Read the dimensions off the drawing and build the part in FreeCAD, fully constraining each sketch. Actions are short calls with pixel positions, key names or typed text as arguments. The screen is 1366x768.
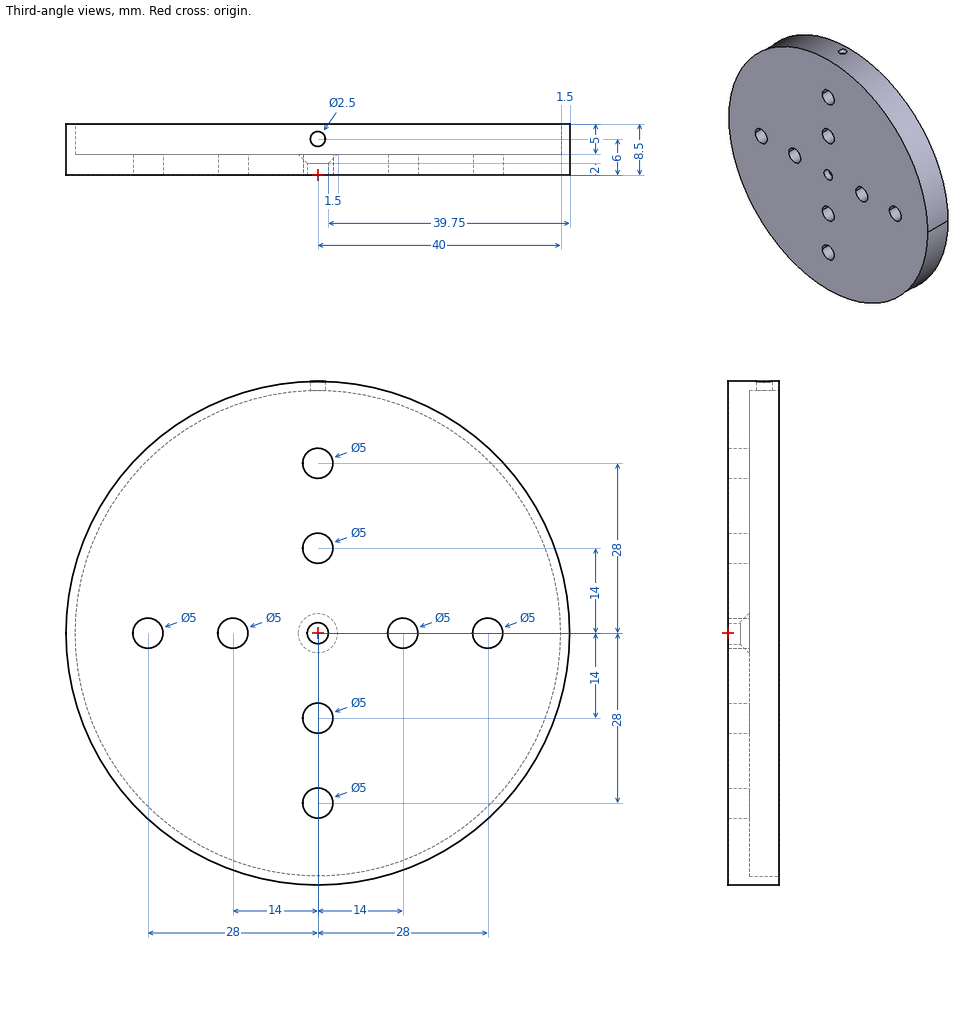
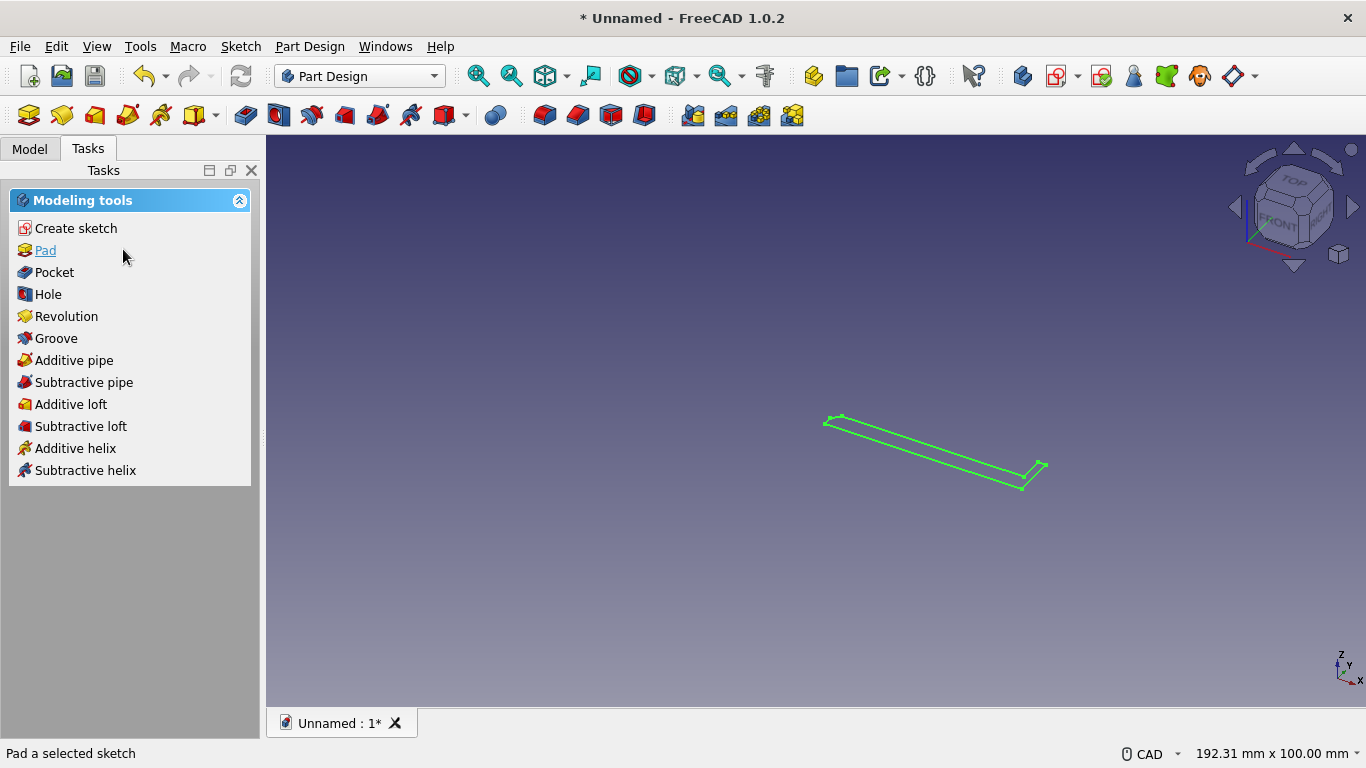
click(62, 116)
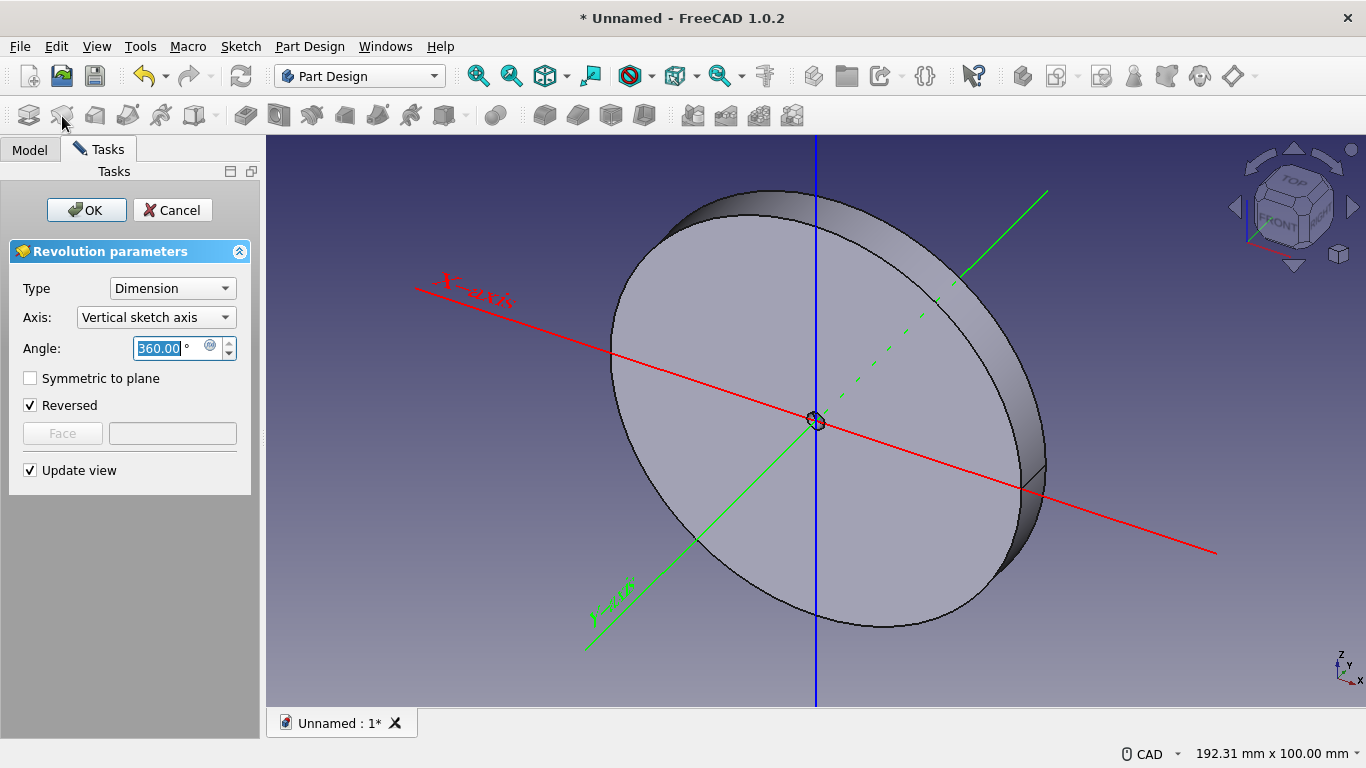
click(87, 210)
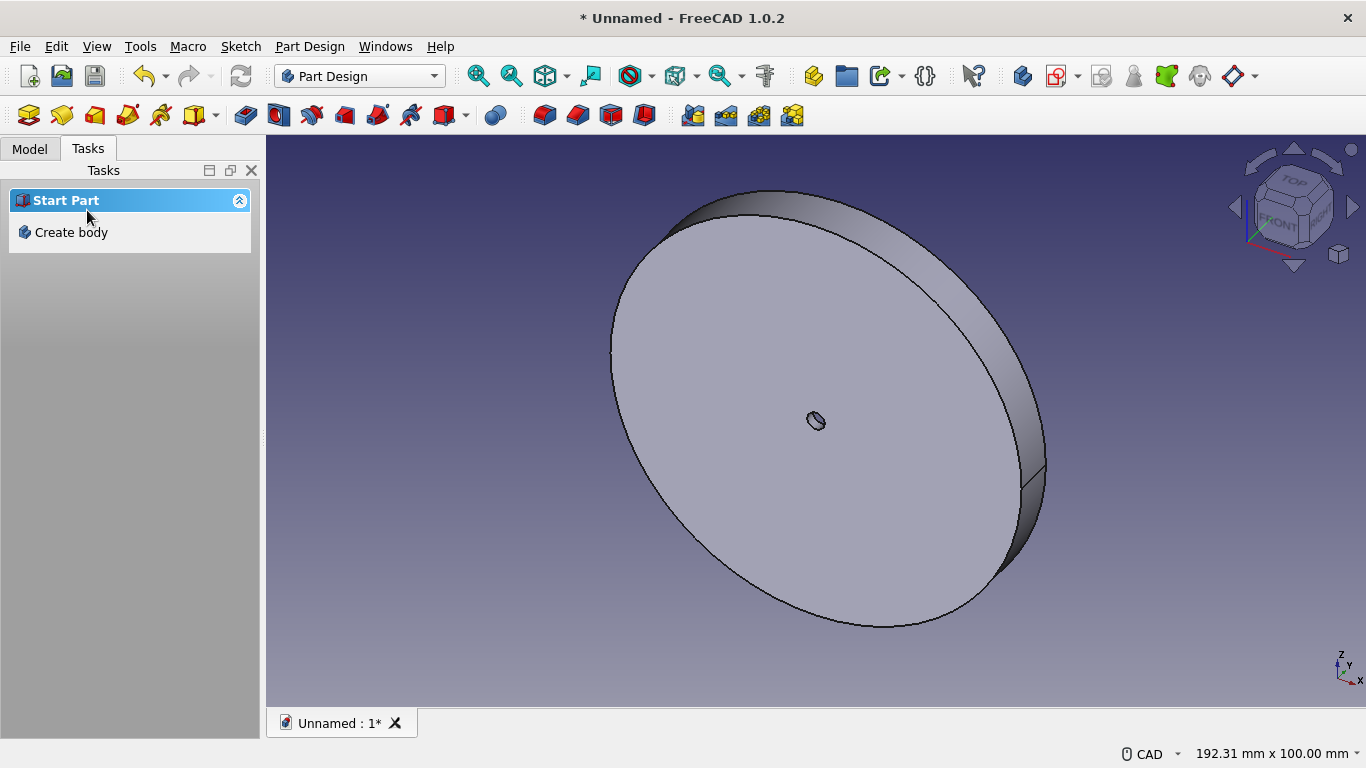
click(479, 76)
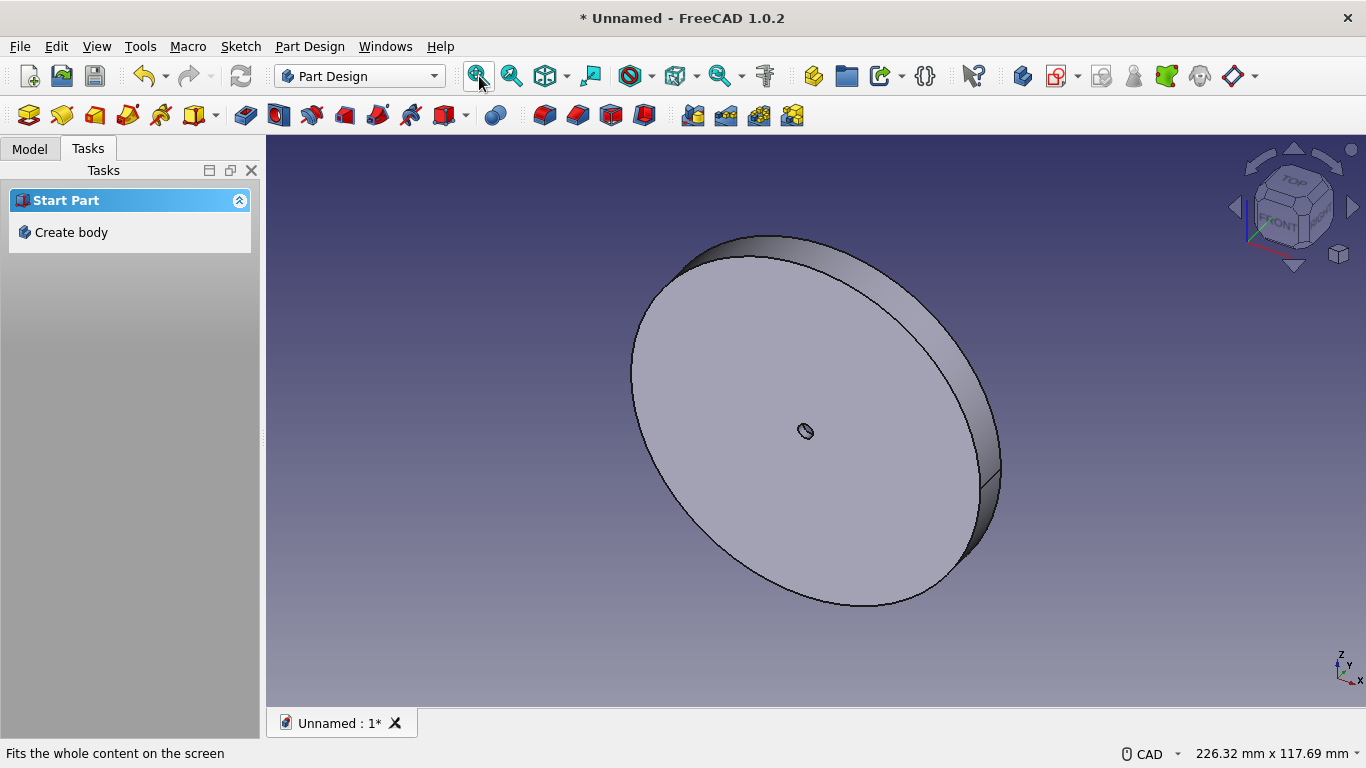
key(4)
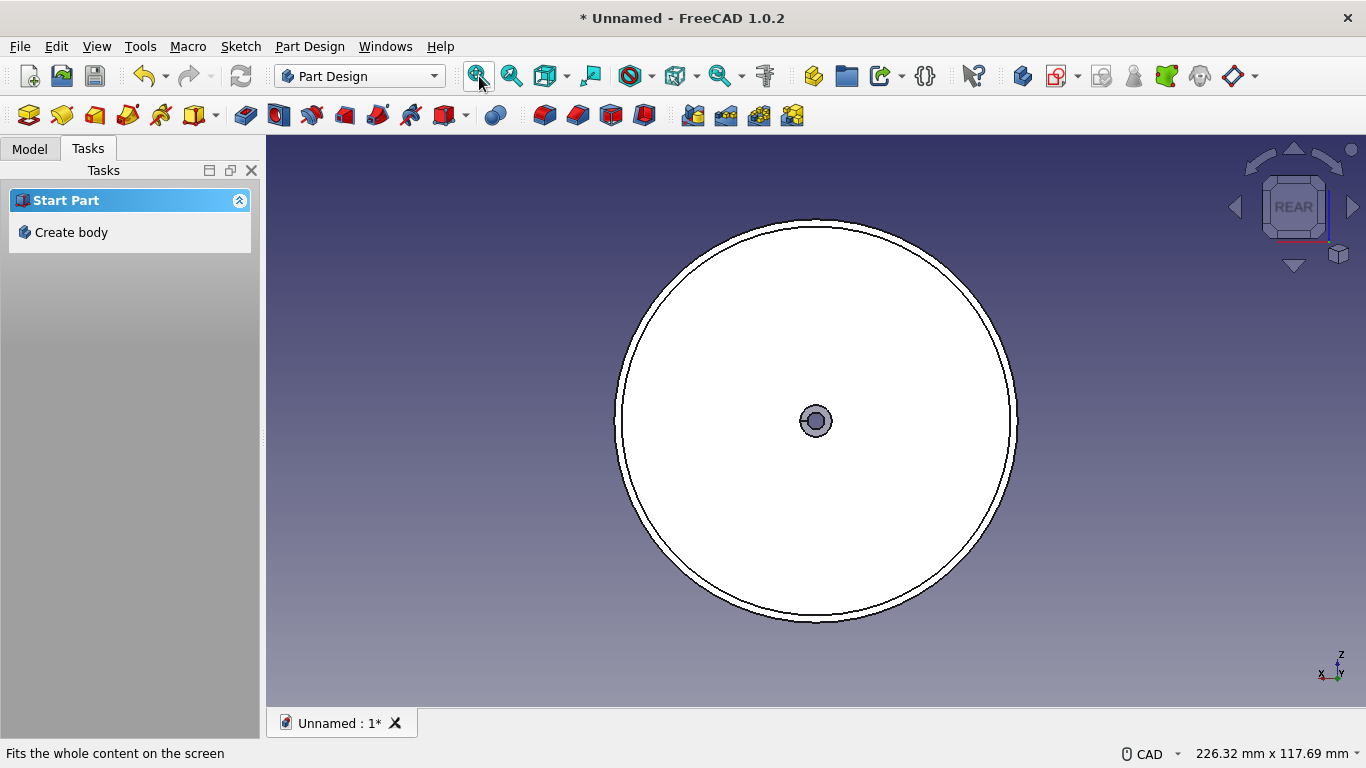
click(705, 420)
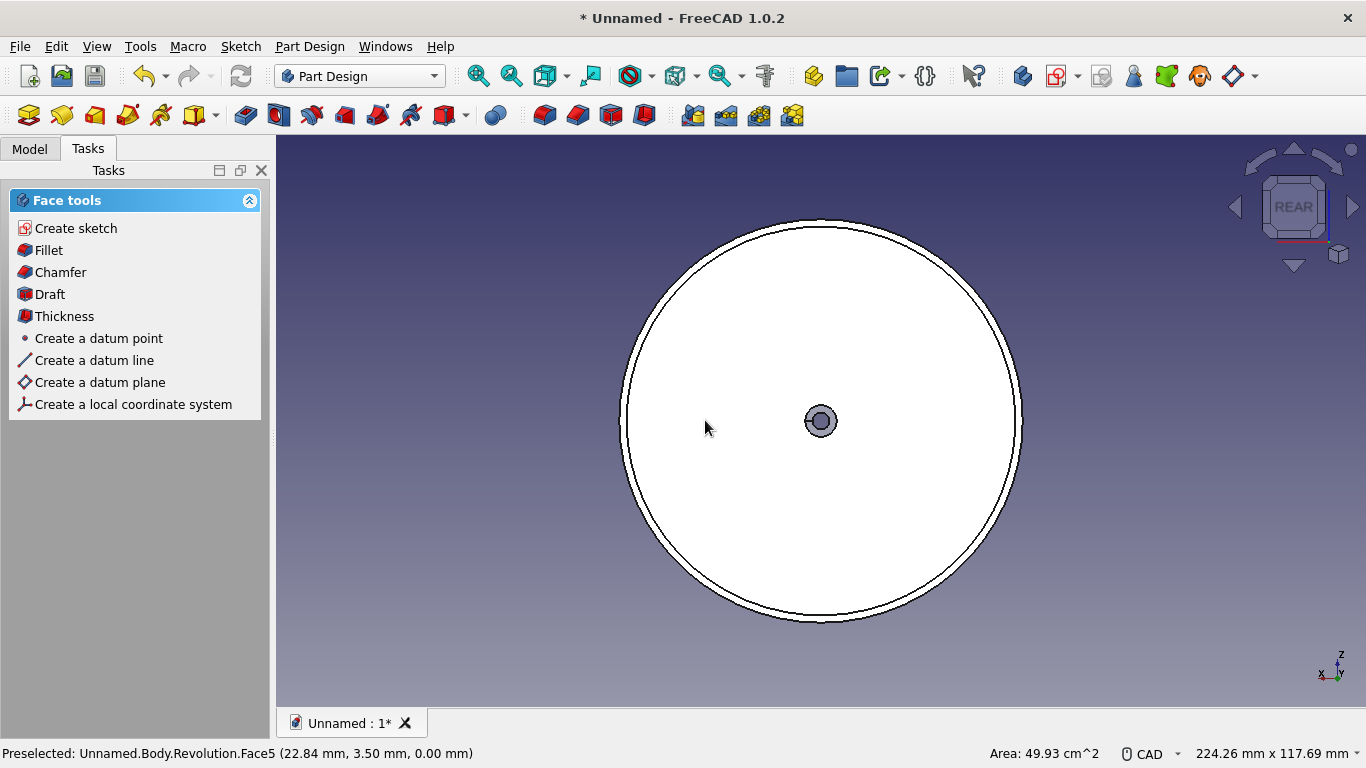
click(1056, 76)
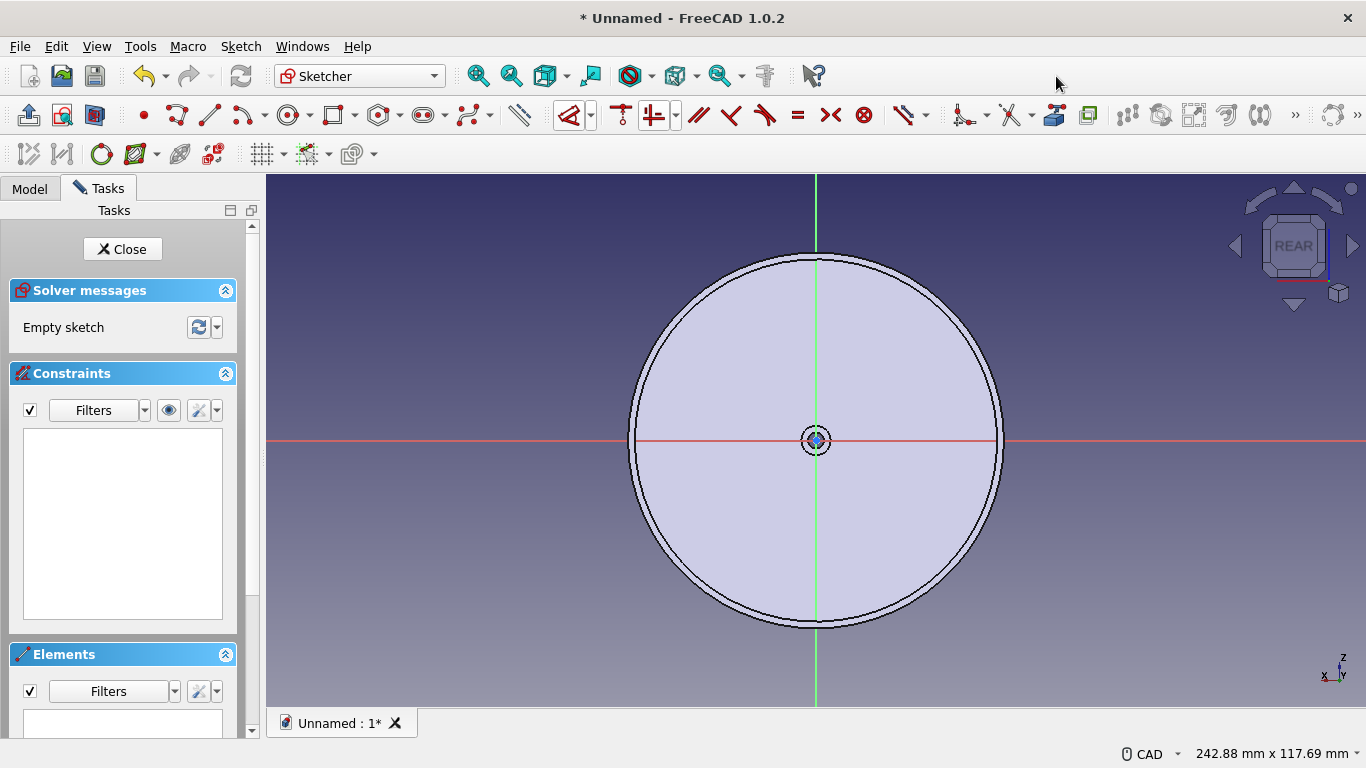
click(95, 116)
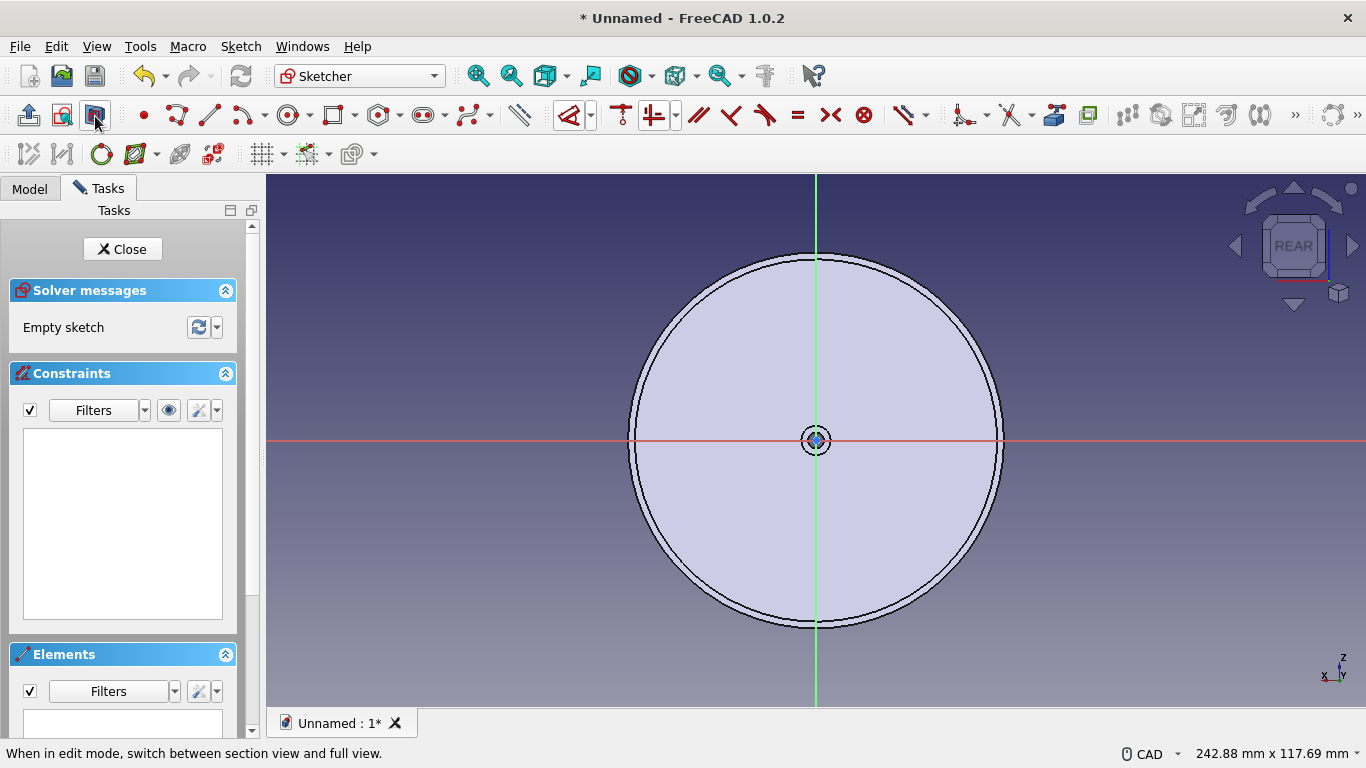
scroll(821, 509, up, 13)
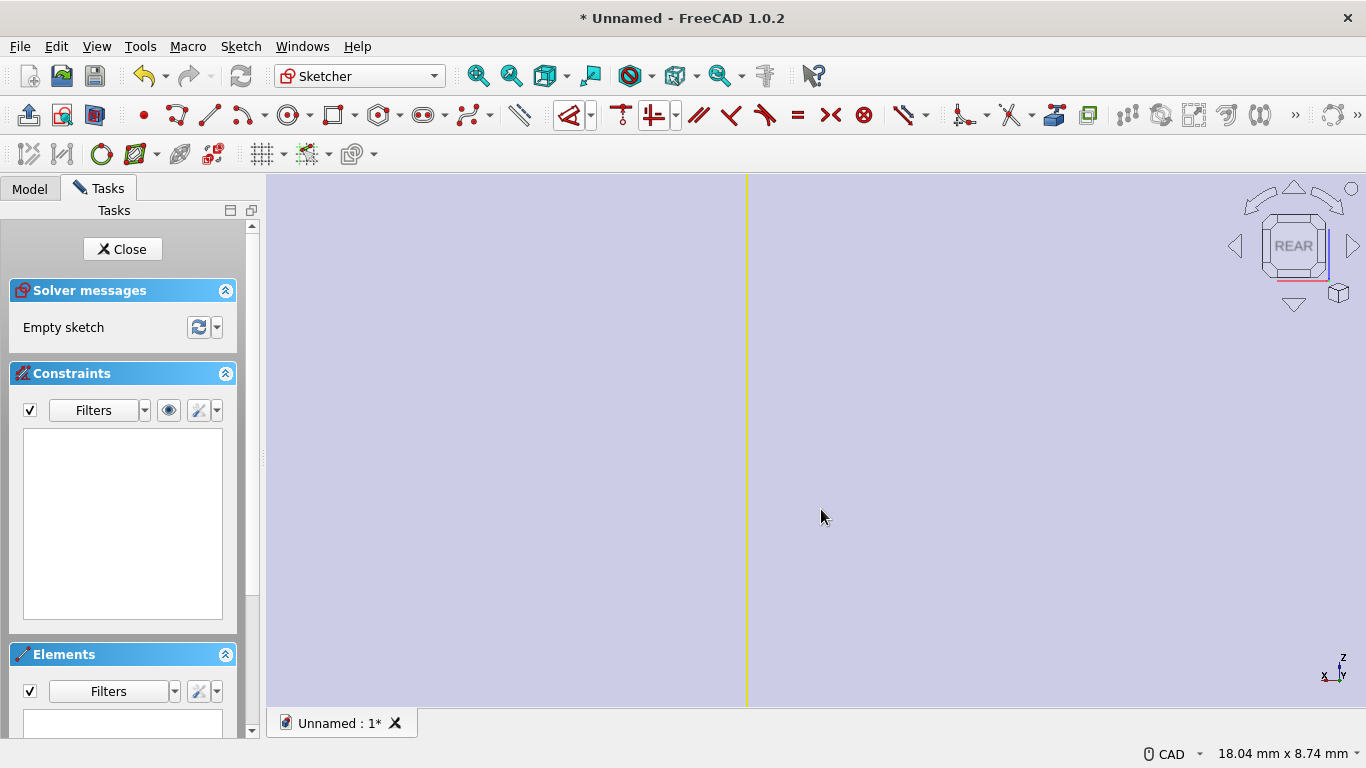
click(288, 116)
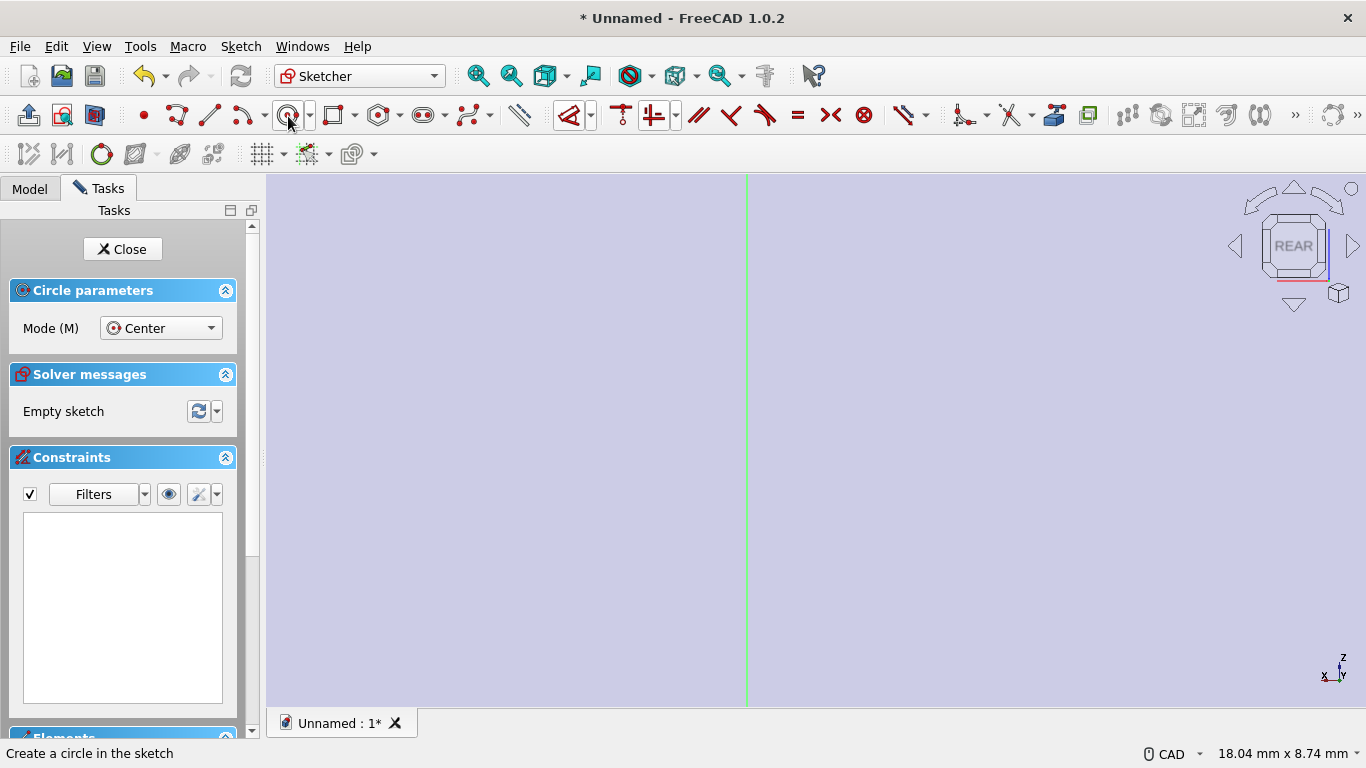
click(747, 433)
click(855, 325)
key(Escape)